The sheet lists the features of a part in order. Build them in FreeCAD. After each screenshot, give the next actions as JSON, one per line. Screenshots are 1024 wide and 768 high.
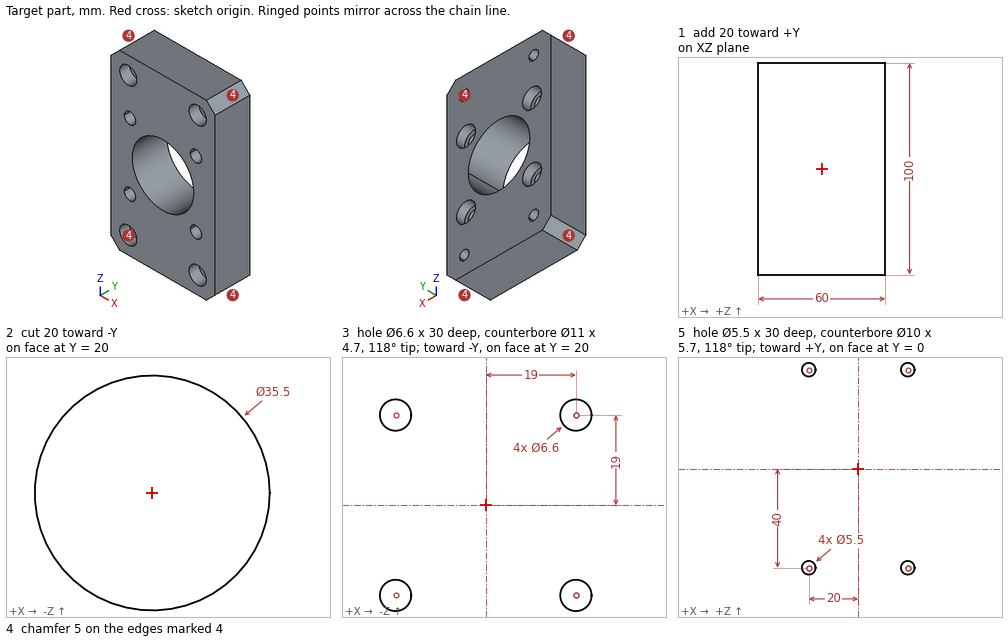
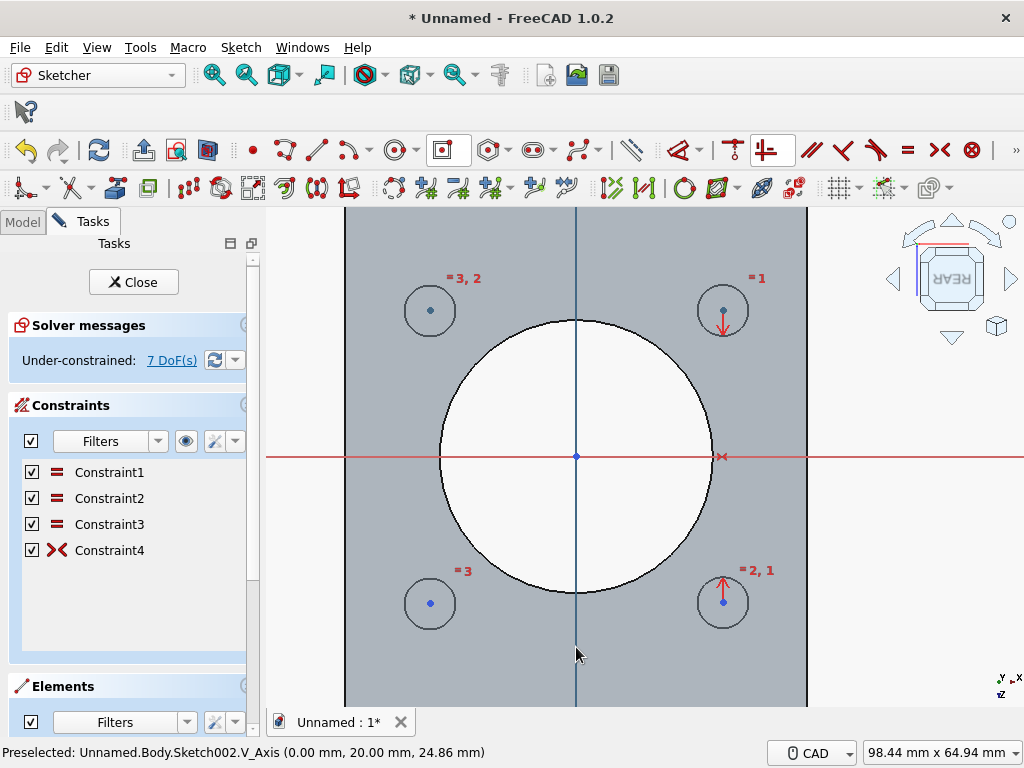
{"action": "key", "text": "s"}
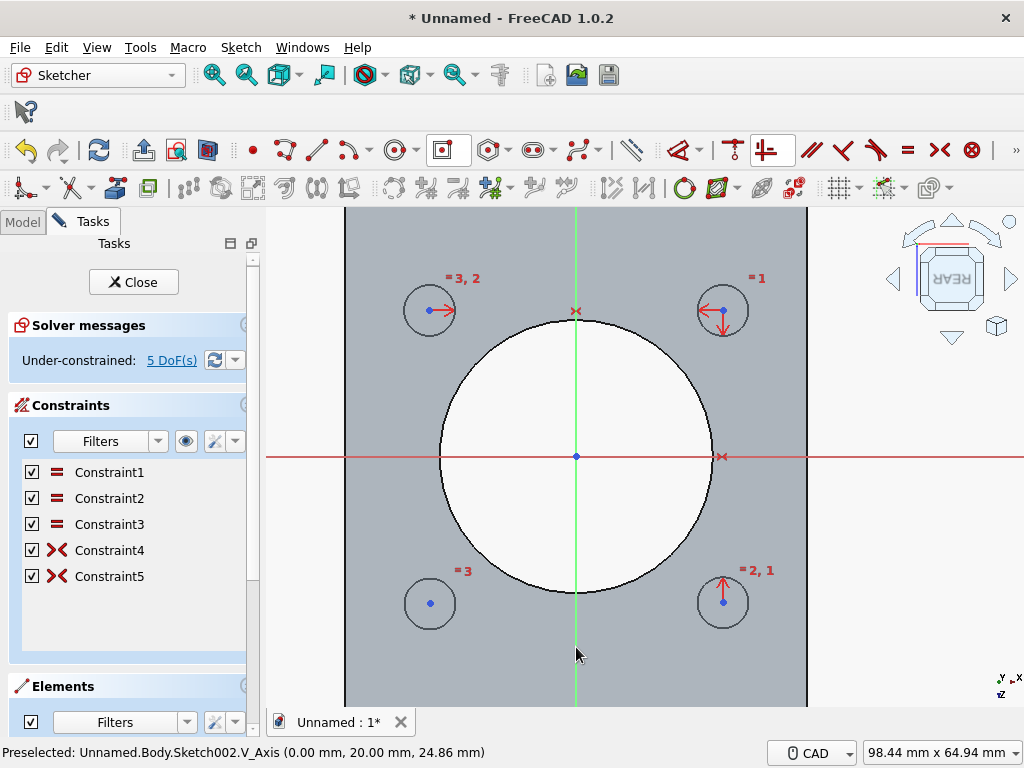
{"action": "left_click", "coordinate": [723, 603]}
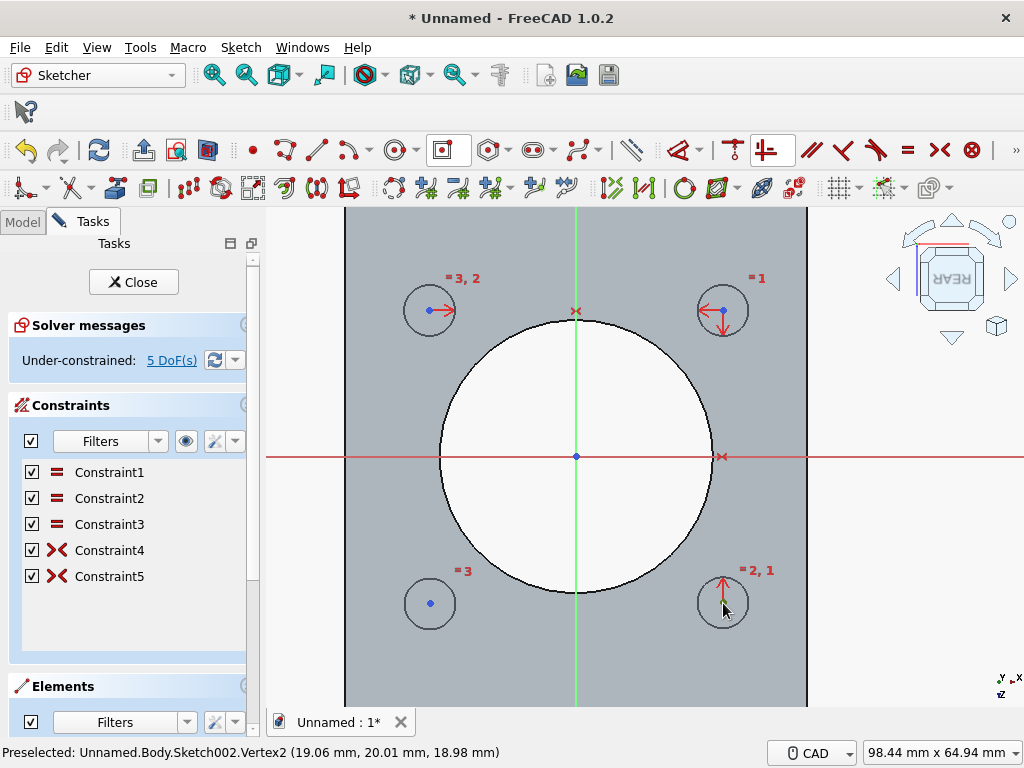
{"action": "left_click", "coordinate": [430, 604]}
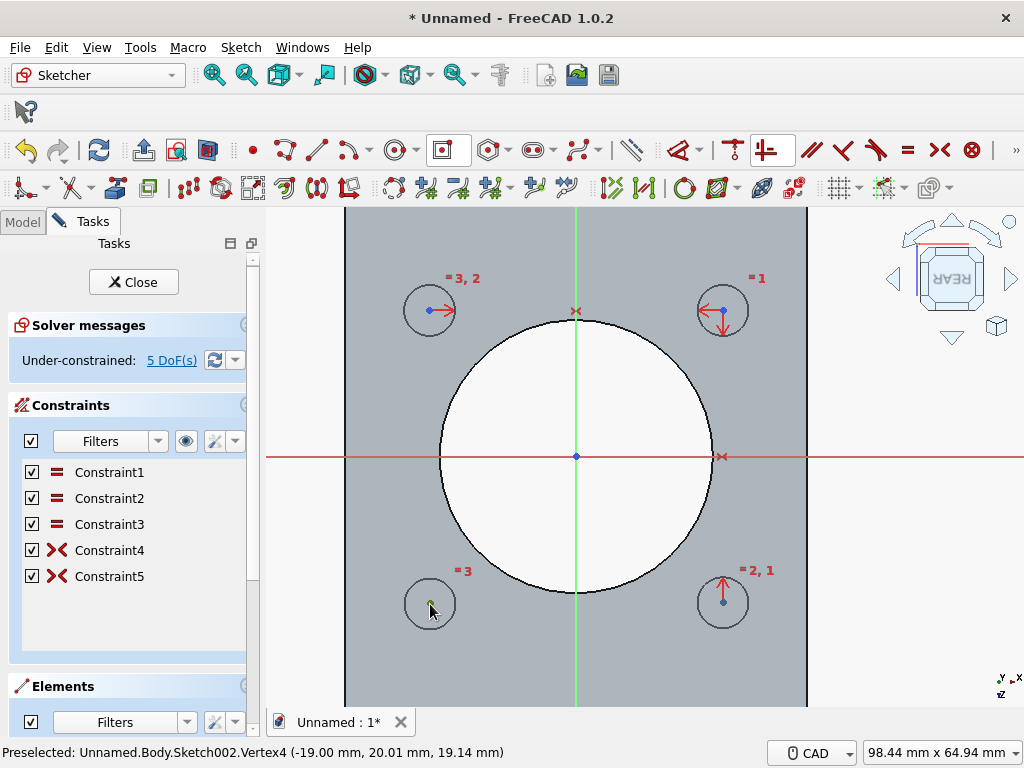
{"action": "left_click", "coordinate": [576, 647]}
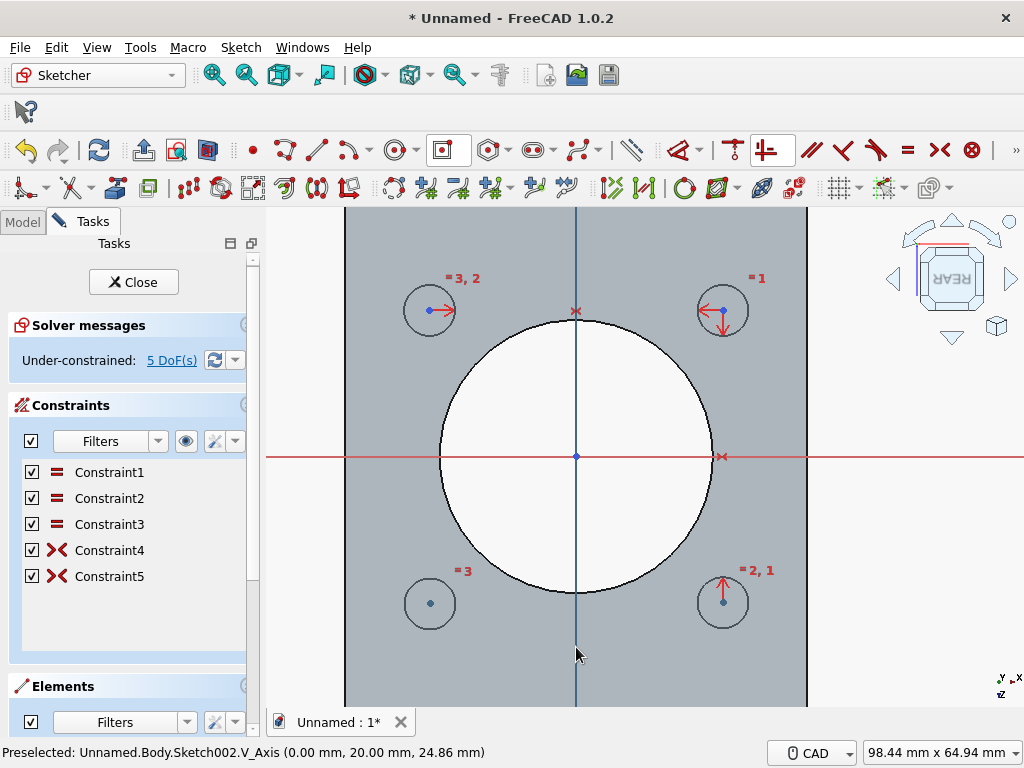
{"action": "key", "text": "s"}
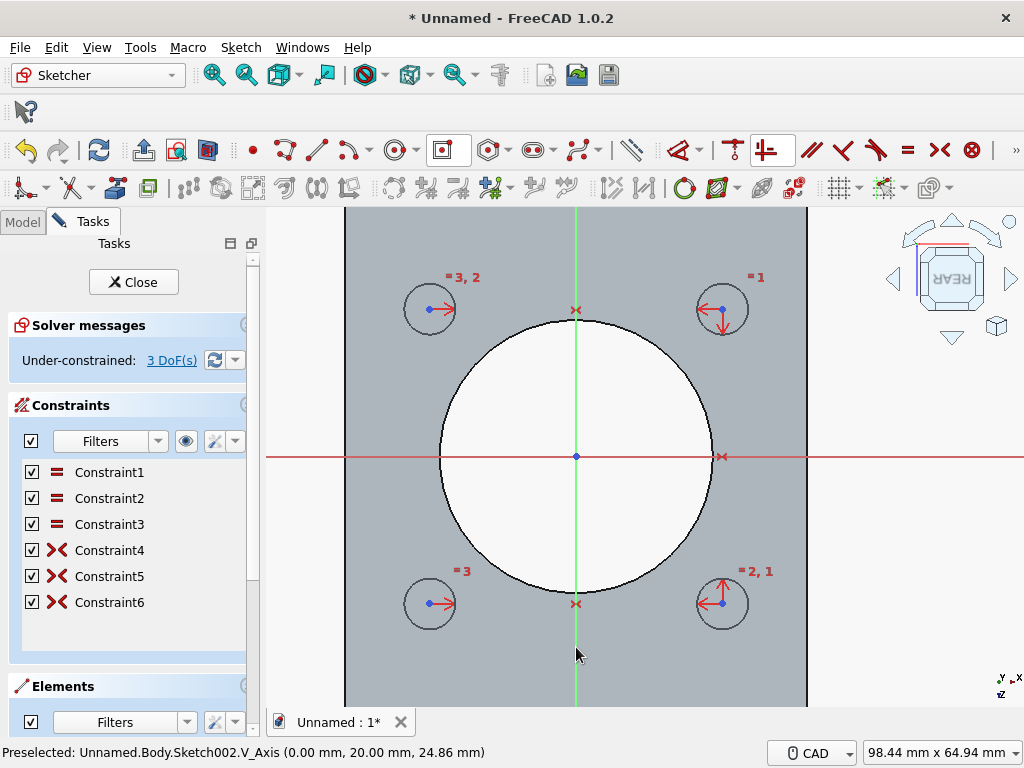
{"action": "left_click", "coordinate": [678, 150]}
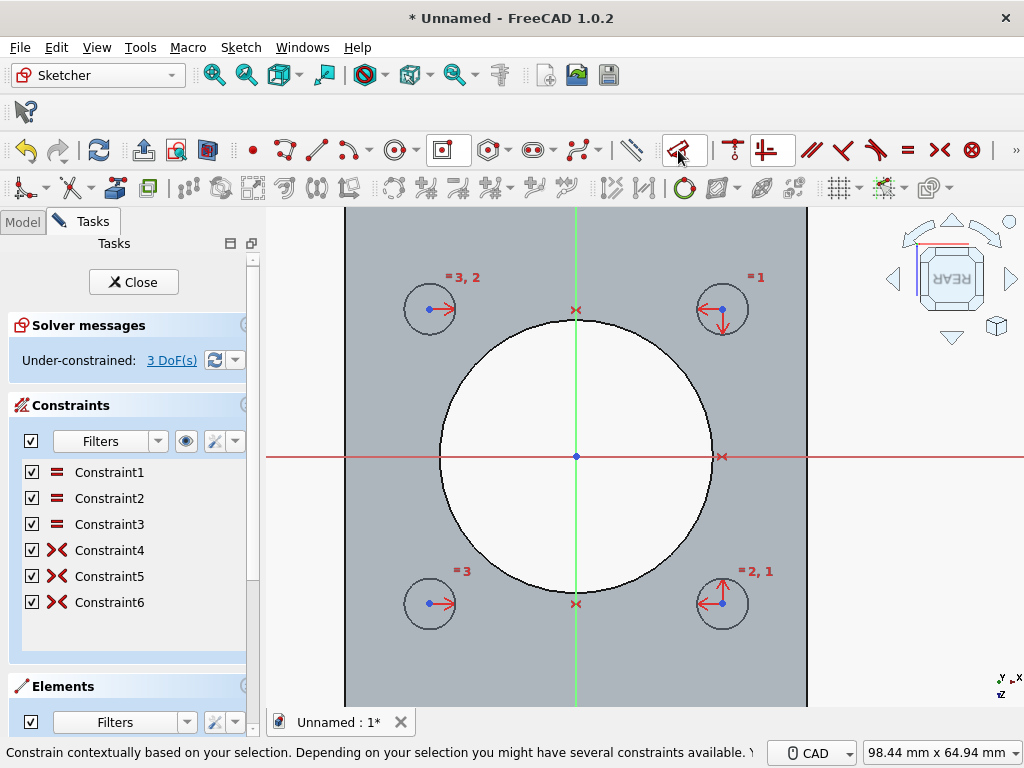
{"action": "left_click", "coordinate": [741, 291]}
{"action": "left_click", "coordinate": [764, 268]}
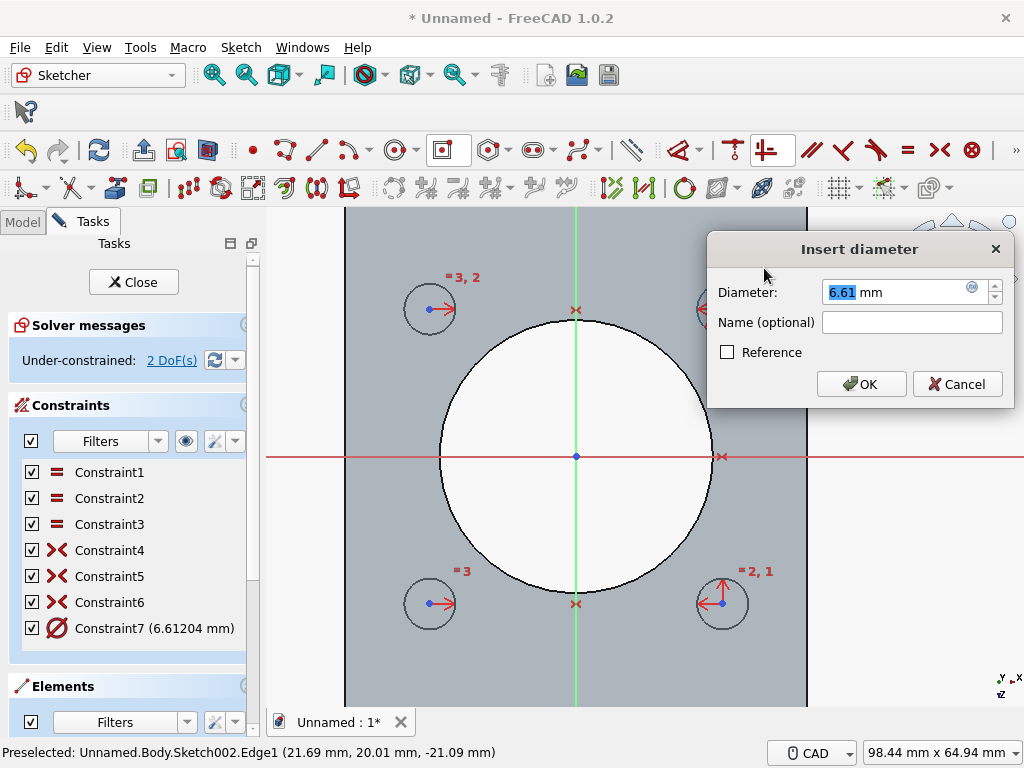
{"action": "type", "text": "6.6"}
{"action": "key", "text": "Return"}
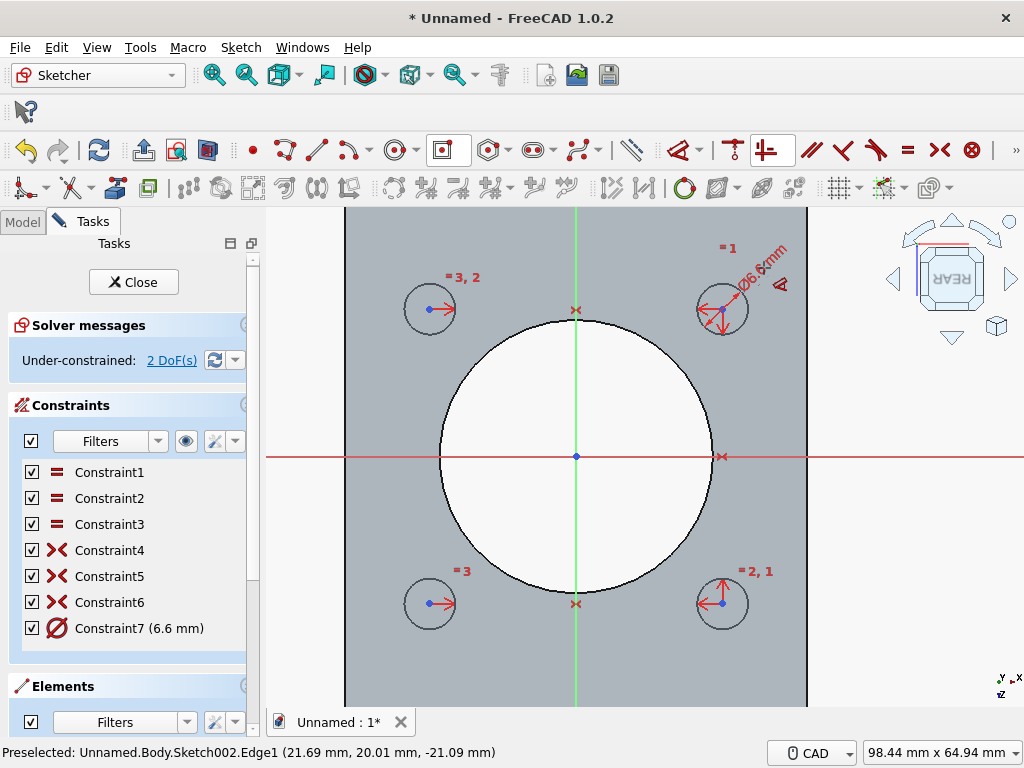
{"action": "left_click", "coordinate": [723, 309]}
{"action": "left_click", "coordinate": [649, 275]}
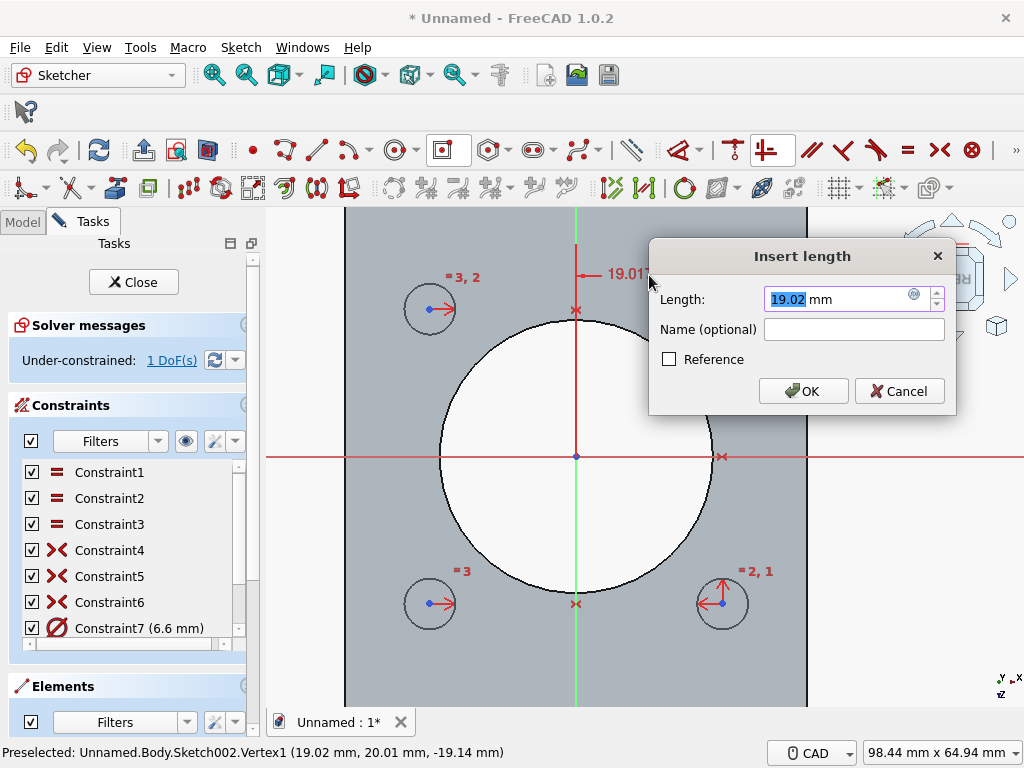
{"action": "type", "text": "19"}
{"action": "key", "text": "Return"}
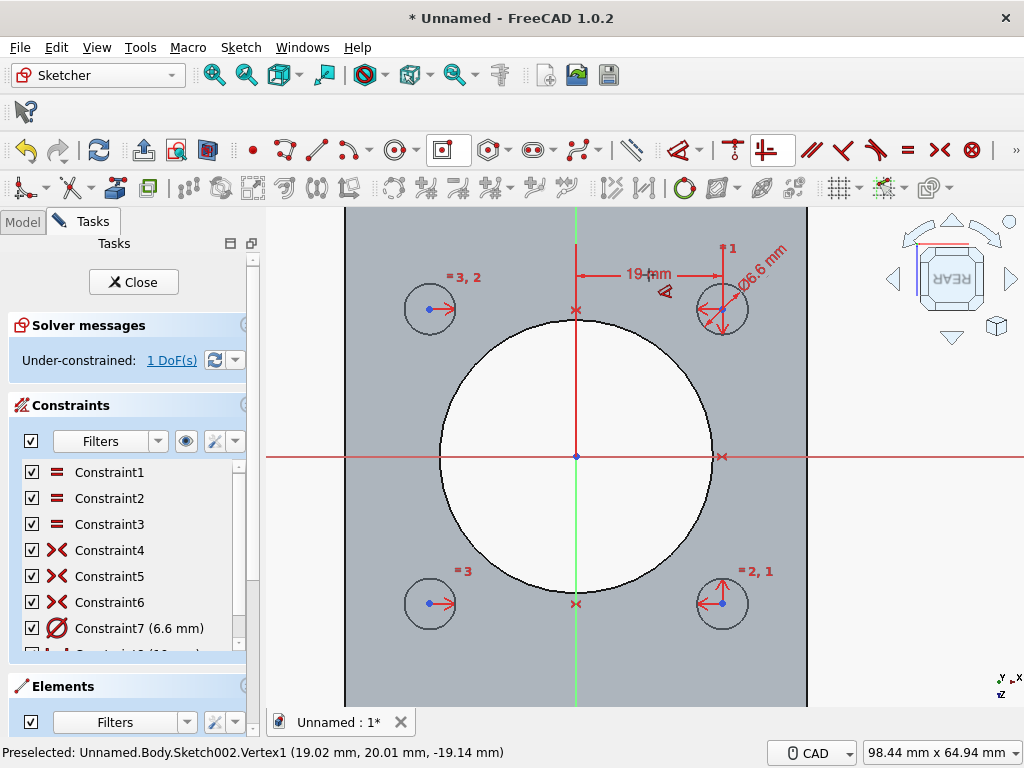
{"action": "left_click", "coordinate": [723, 309]}
{"action": "left_click", "coordinate": [757, 383]}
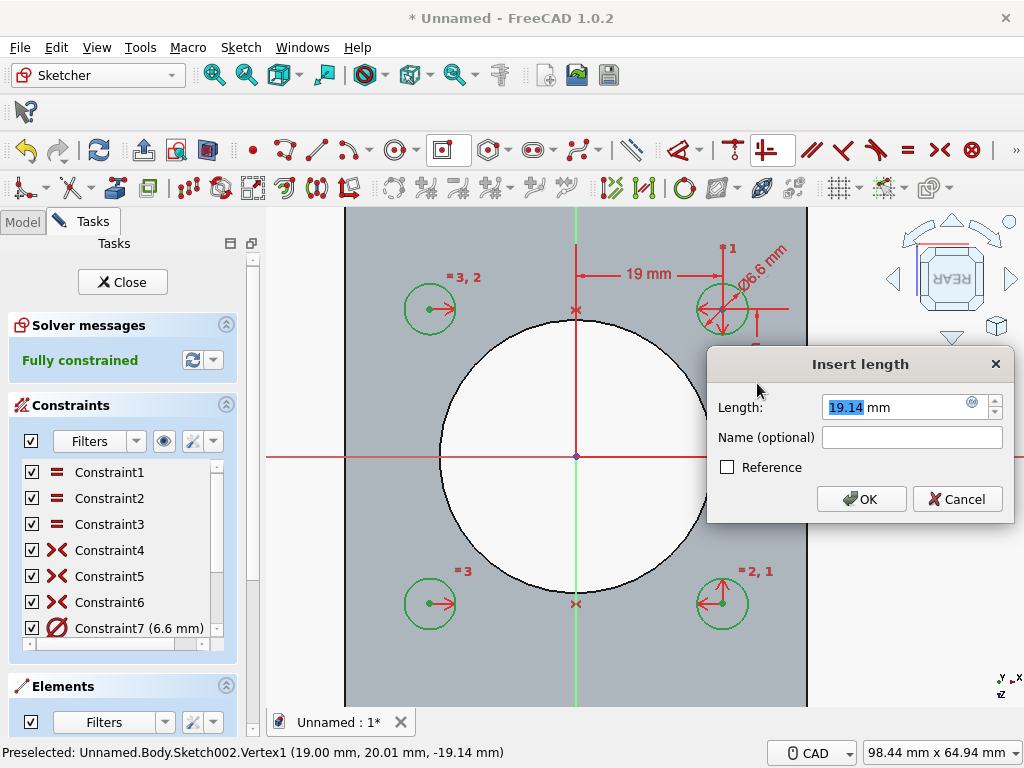
{"action": "type", "text": "19"}
{"action": "key", "text": "Return"}
{"action": "key", "text": "Escape"}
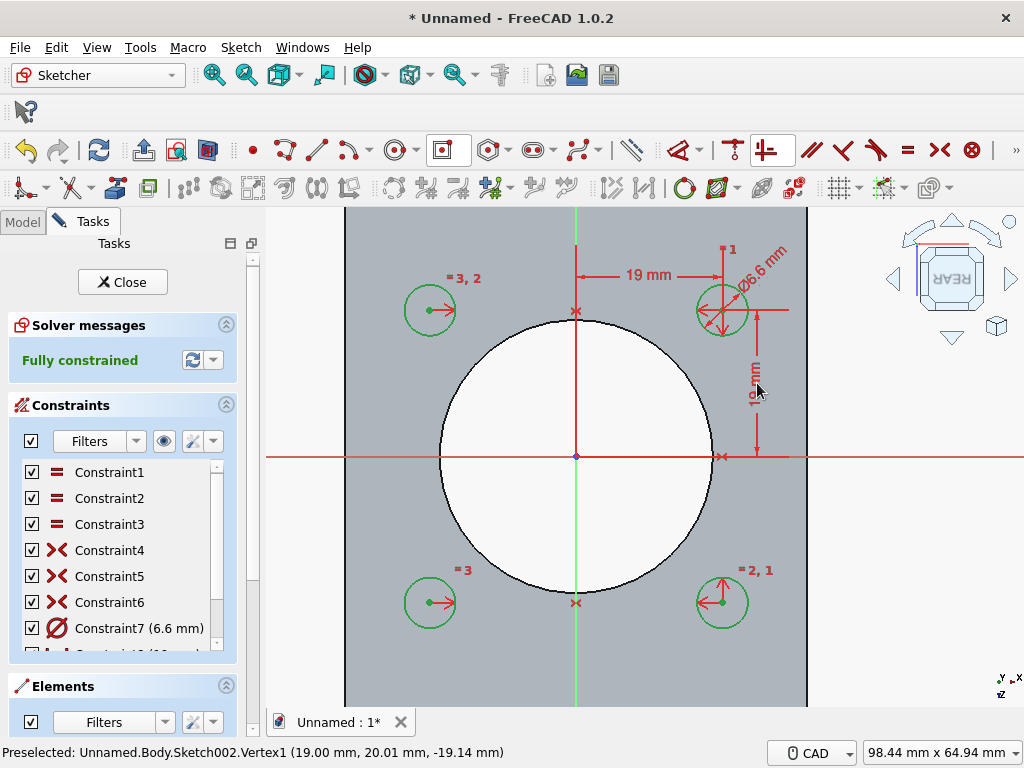
{"action": "left_click", "coordinate": [123, 282]}